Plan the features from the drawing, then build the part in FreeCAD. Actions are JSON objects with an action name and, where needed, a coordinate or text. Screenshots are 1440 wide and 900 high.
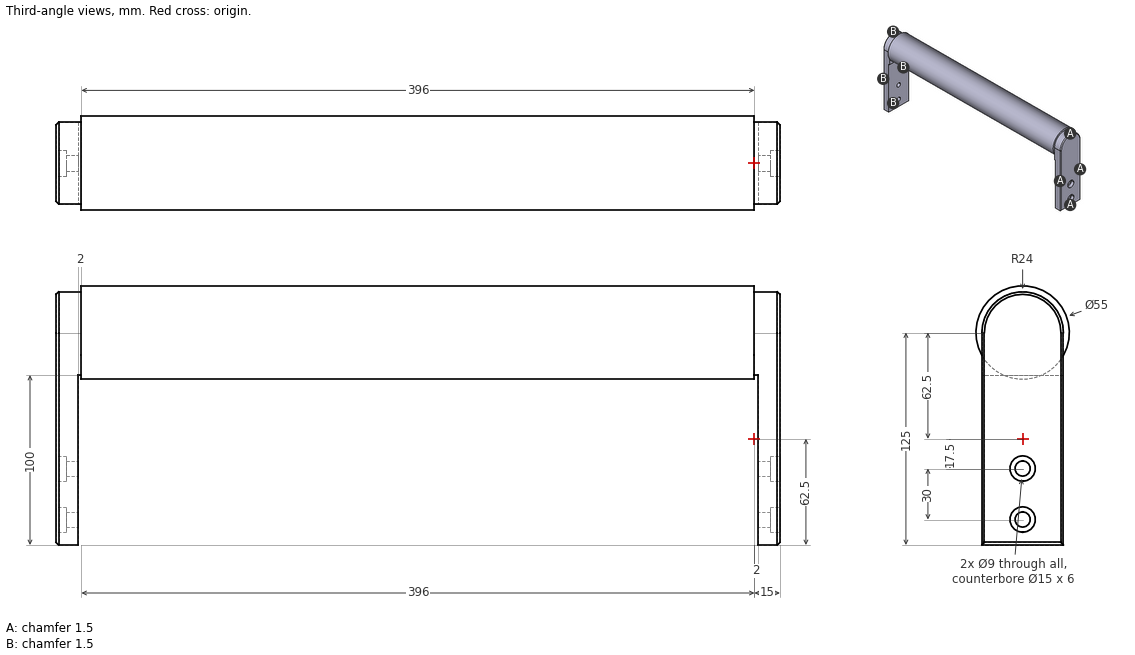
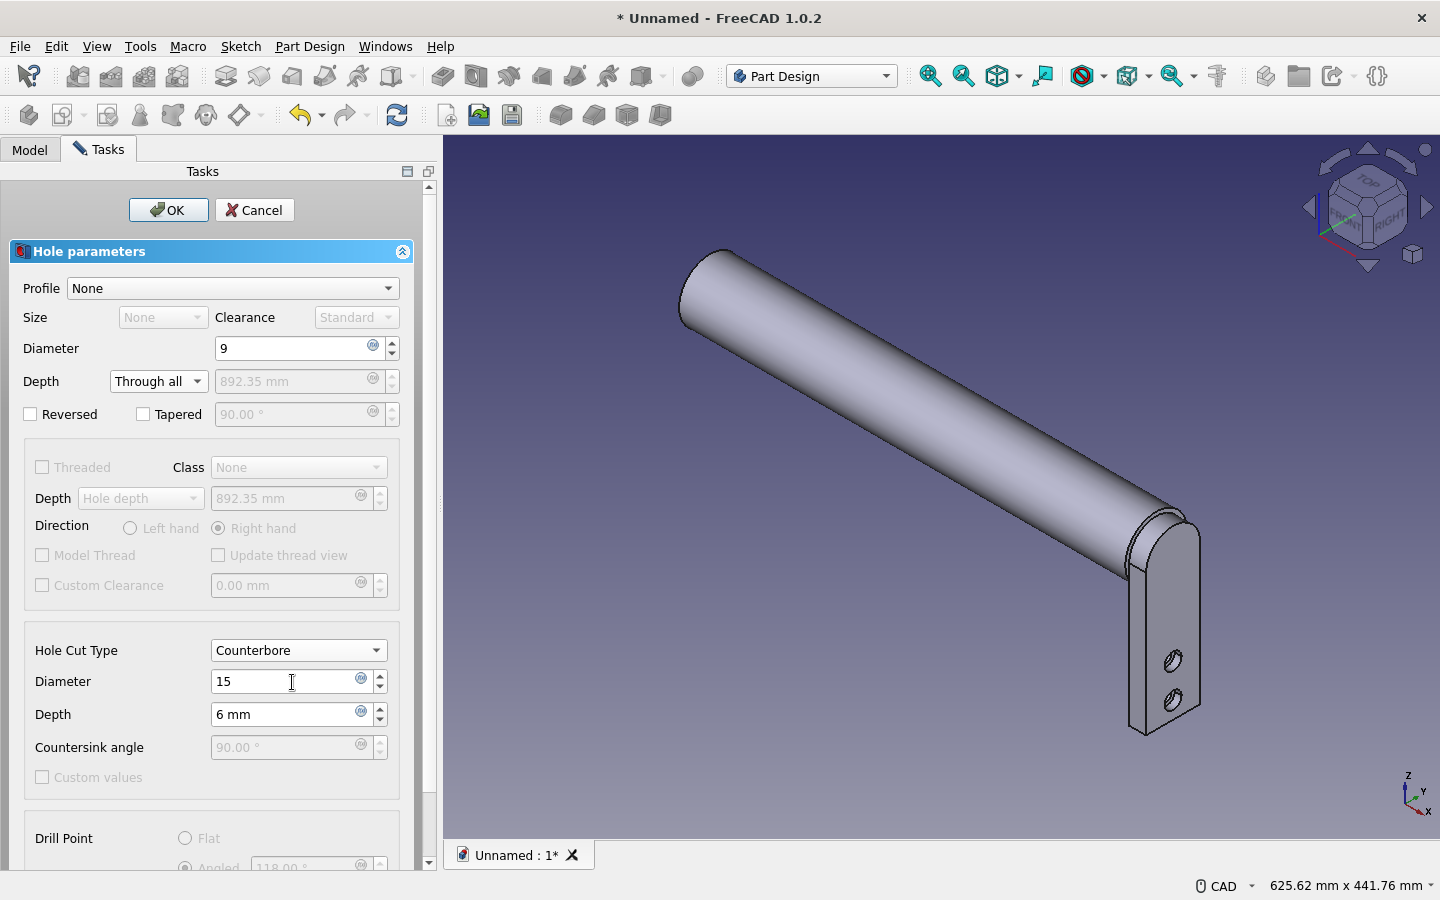
{"action": "left_click", "coordinate": [169, 210]}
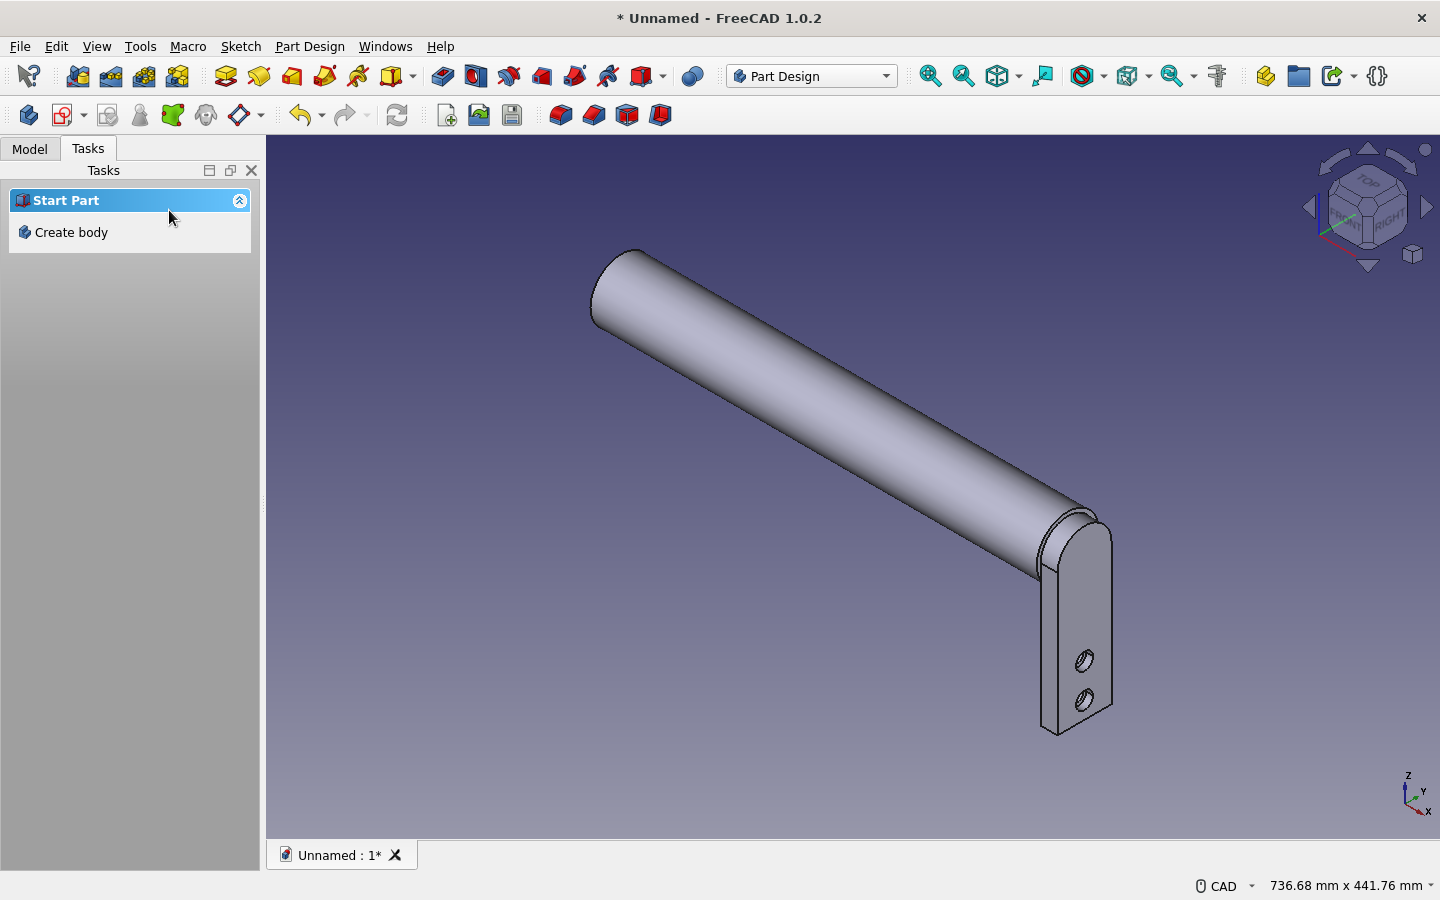
{"action": "left_click", "coordinate": [1085, 525]}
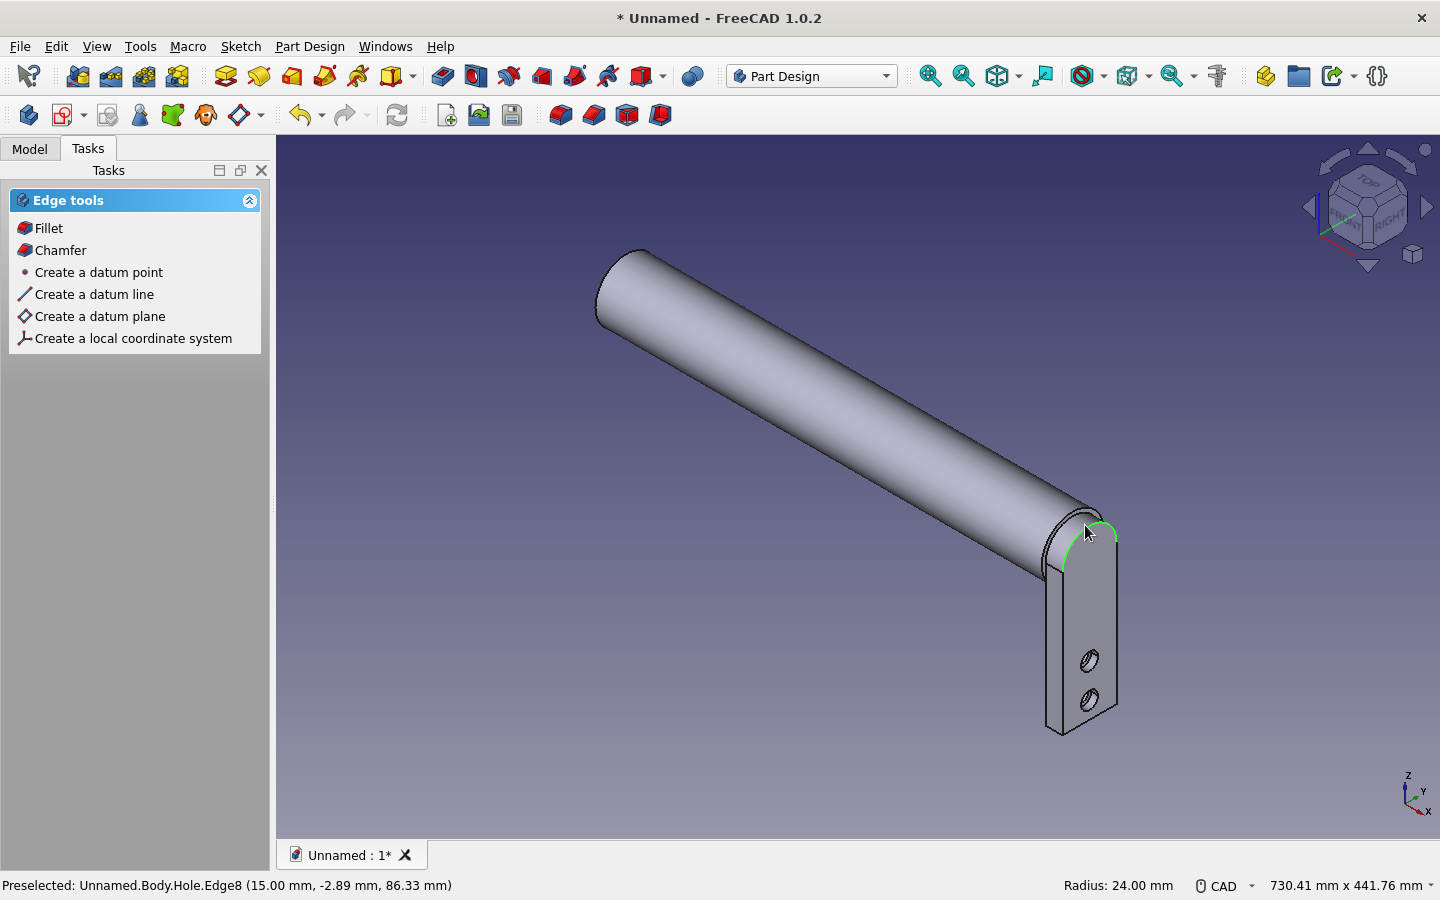
{"action": "left_click", "coordinate": [1063, 653], "text": "ctrl"}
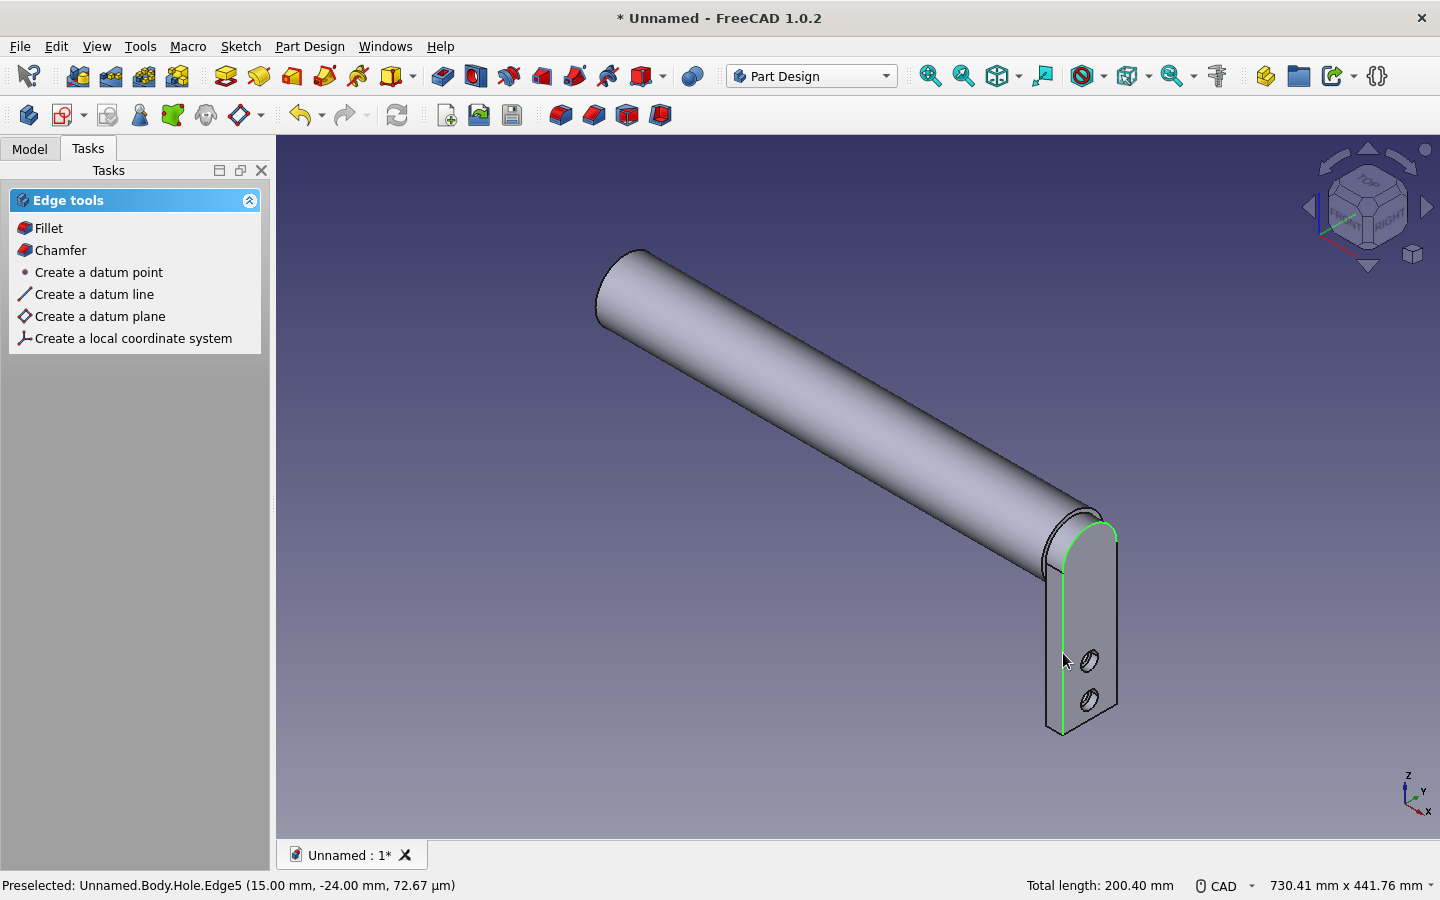
{"action": "key", "text": "2"}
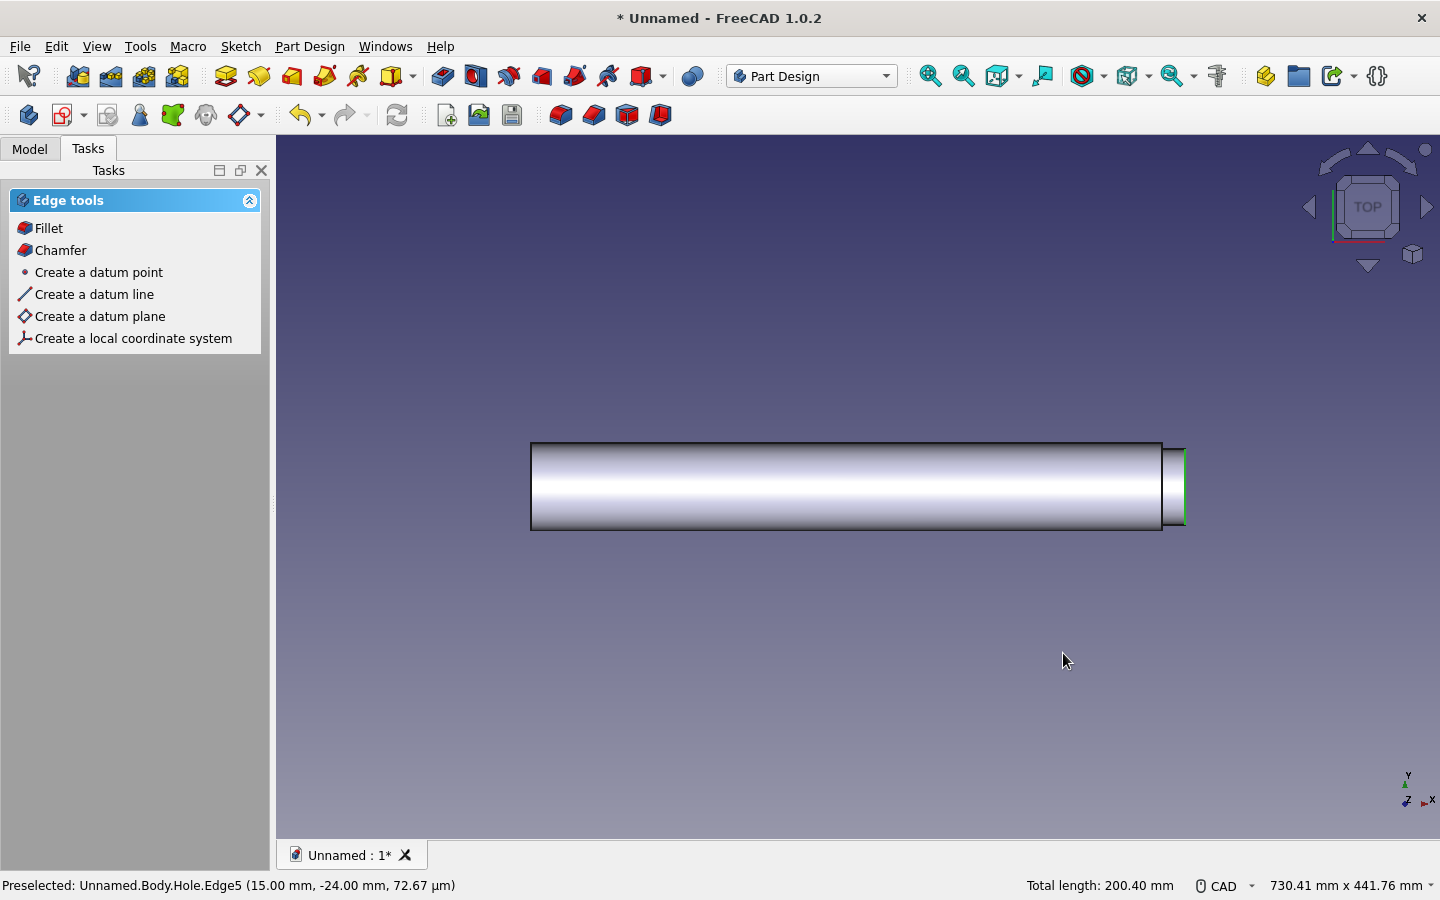
{"action": "key", "text": "0"}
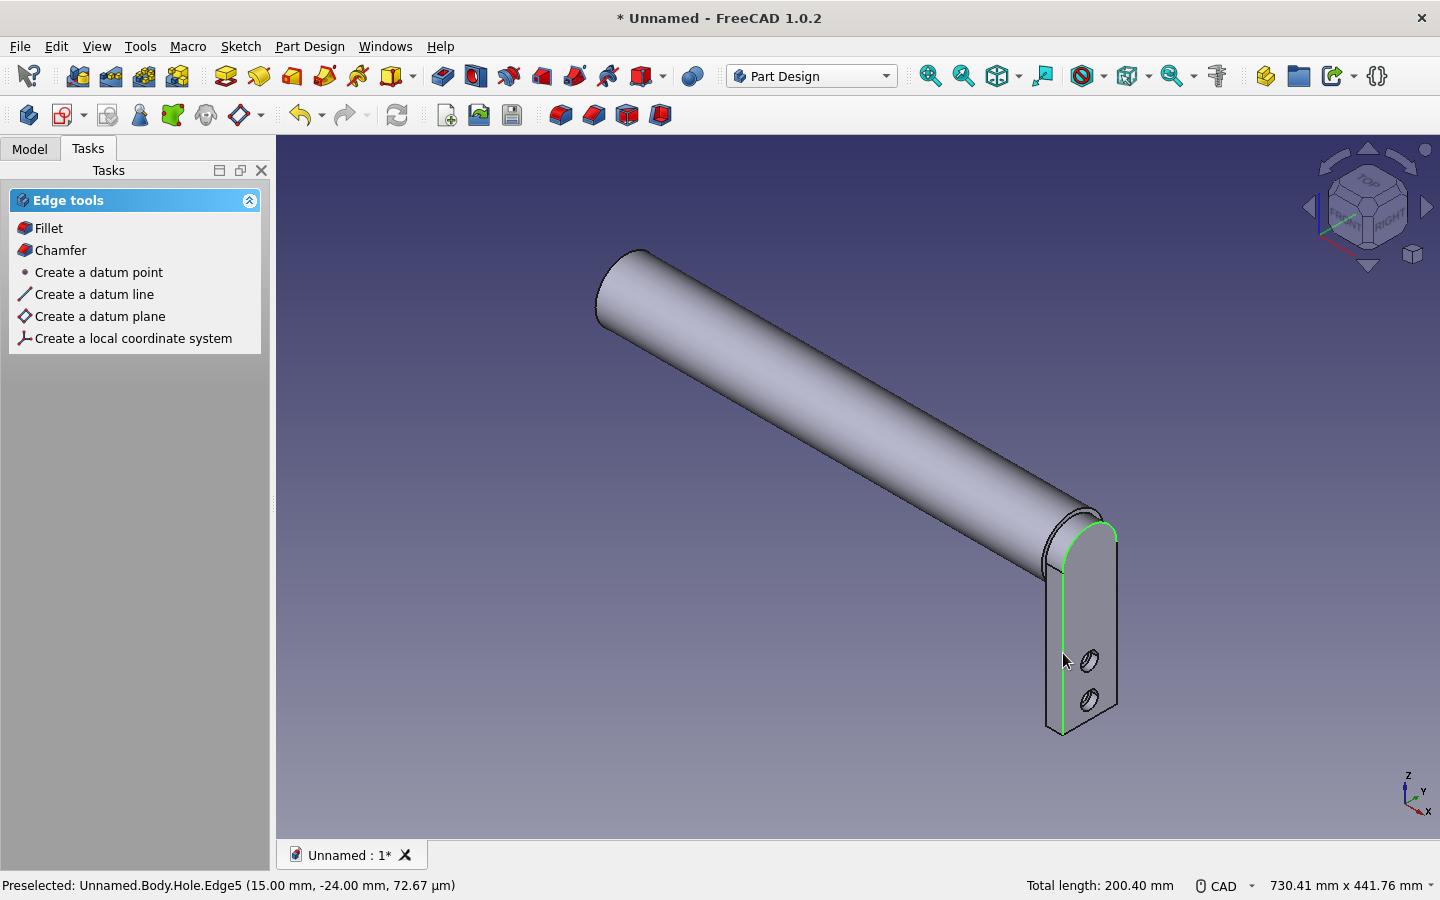
{"action": "key", "text": "1"}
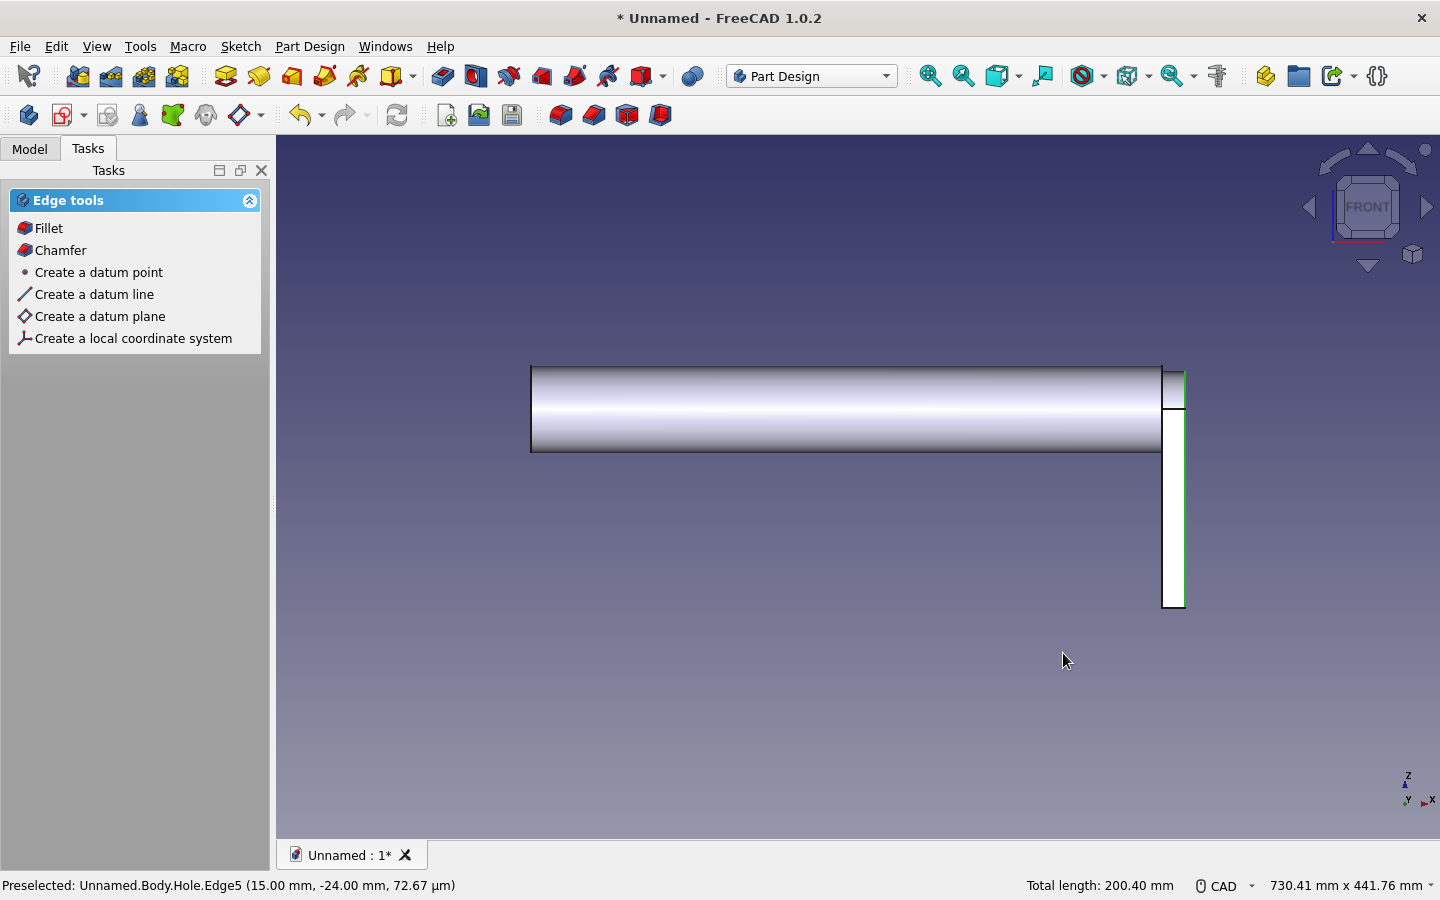
{"action": "key", "text": "3"}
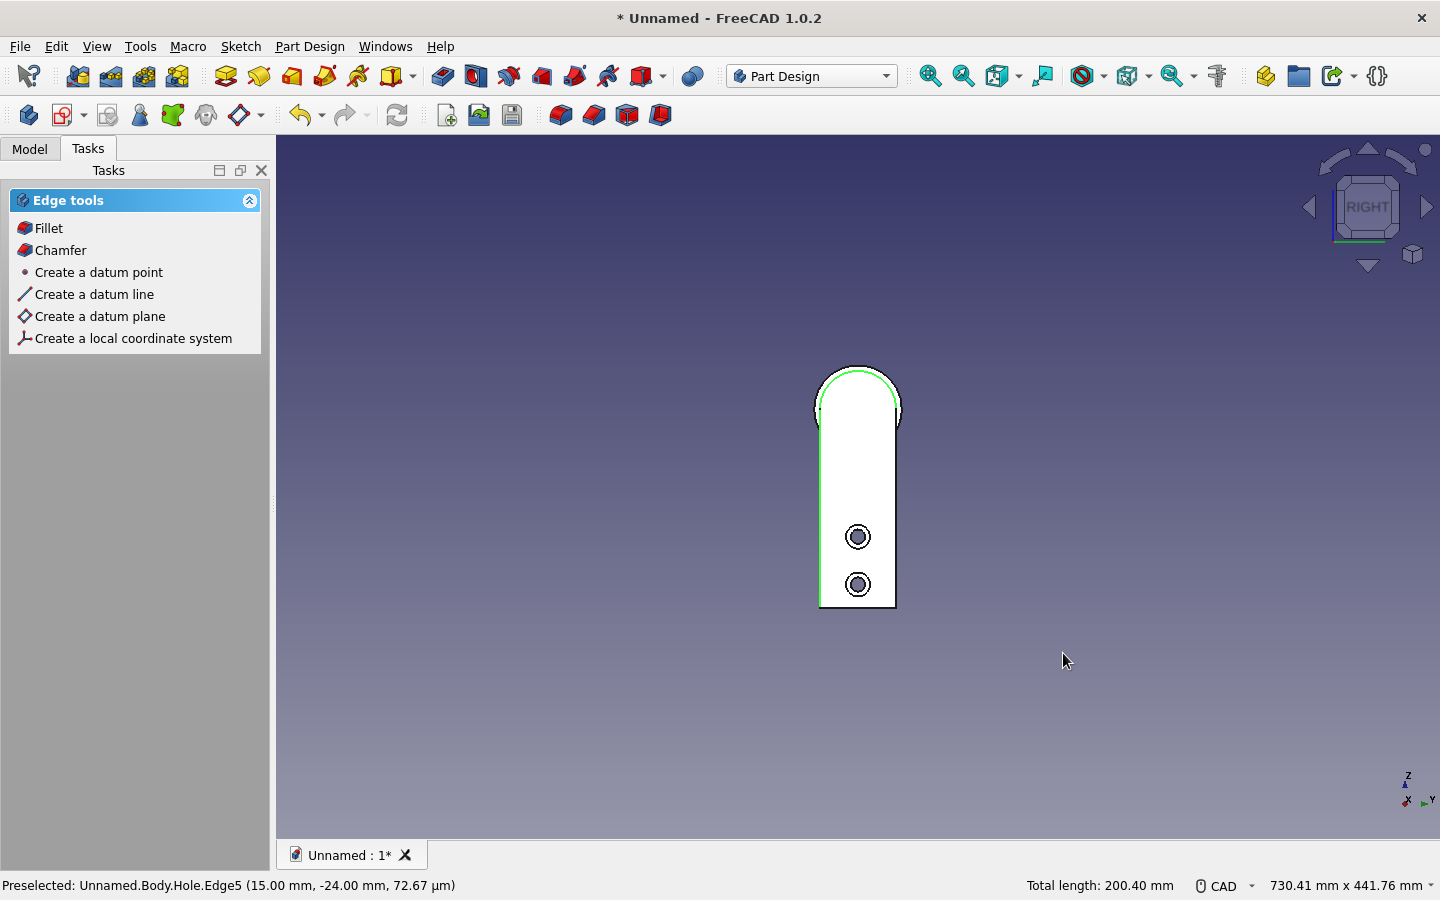
{"action": "left_click", "coordinate": [931, 76]}